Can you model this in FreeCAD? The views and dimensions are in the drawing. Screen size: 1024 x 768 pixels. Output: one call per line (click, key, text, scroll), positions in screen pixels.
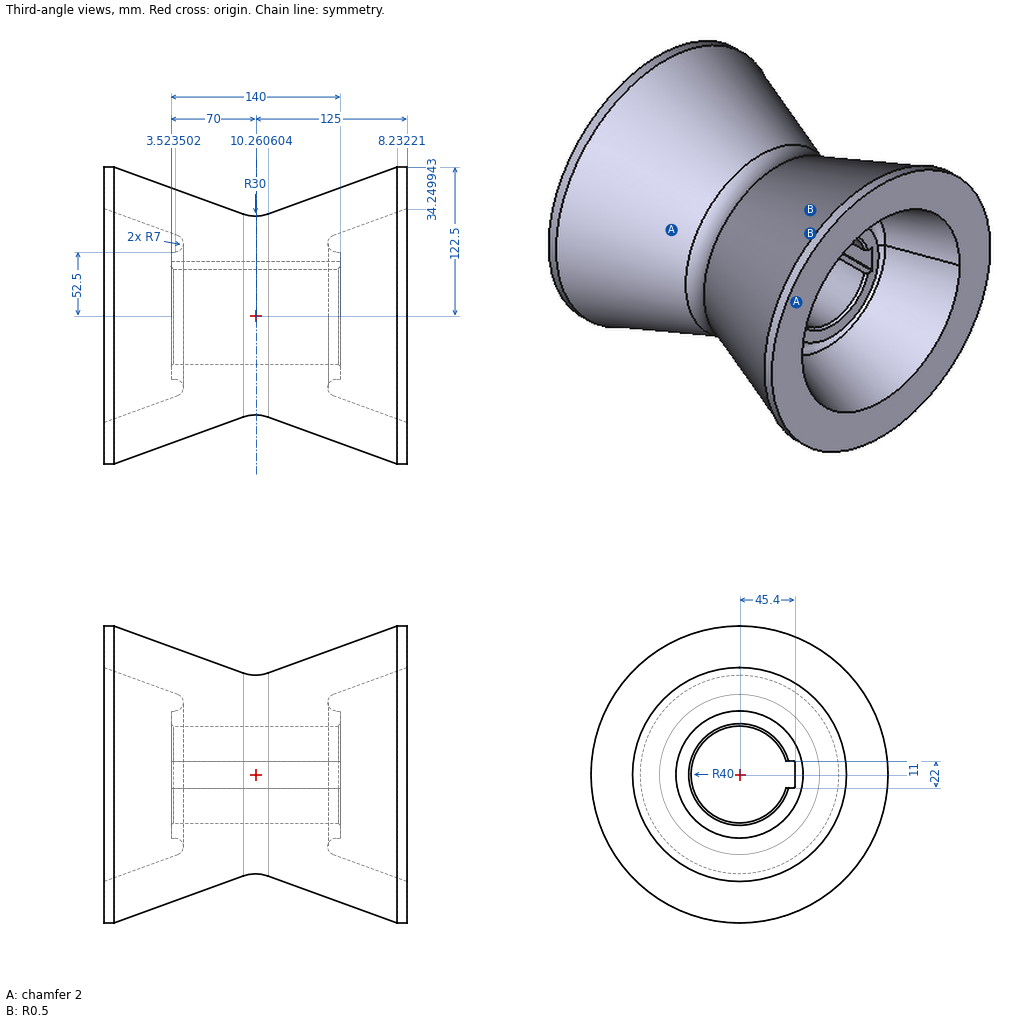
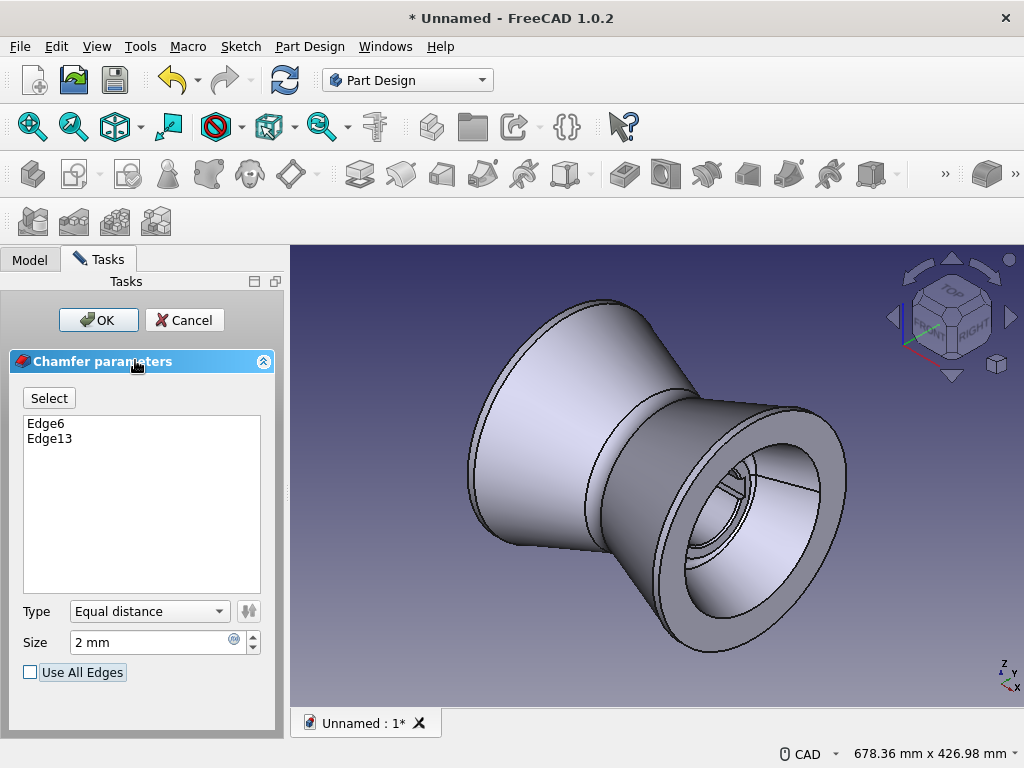
click(99, 320)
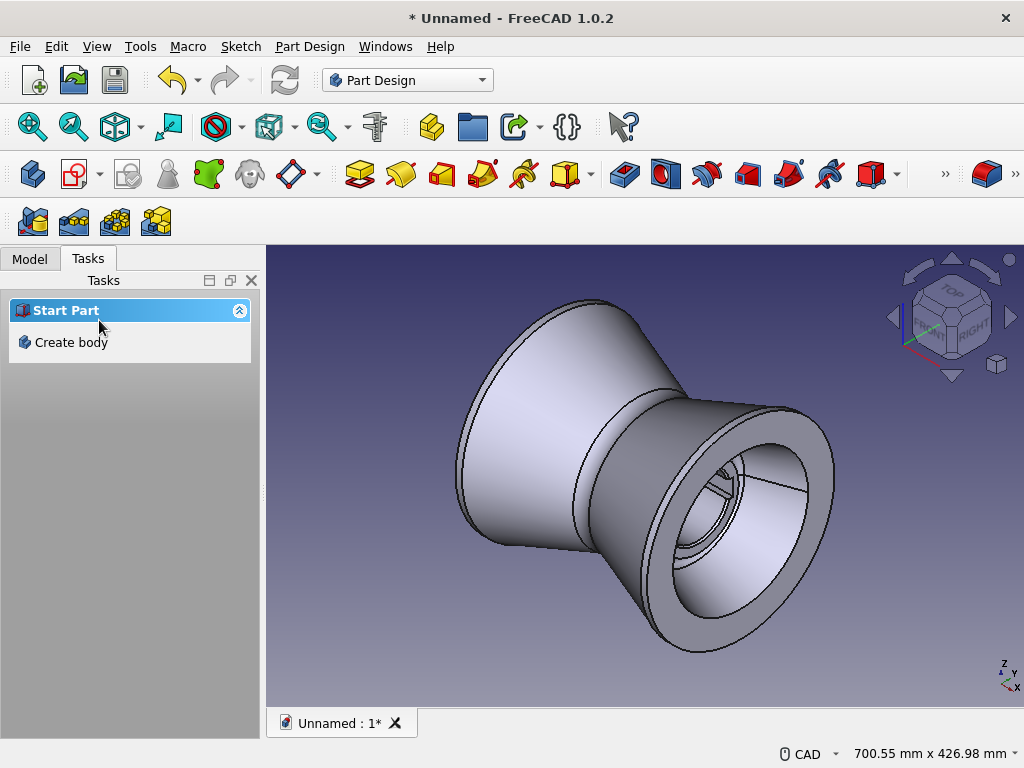
key(2)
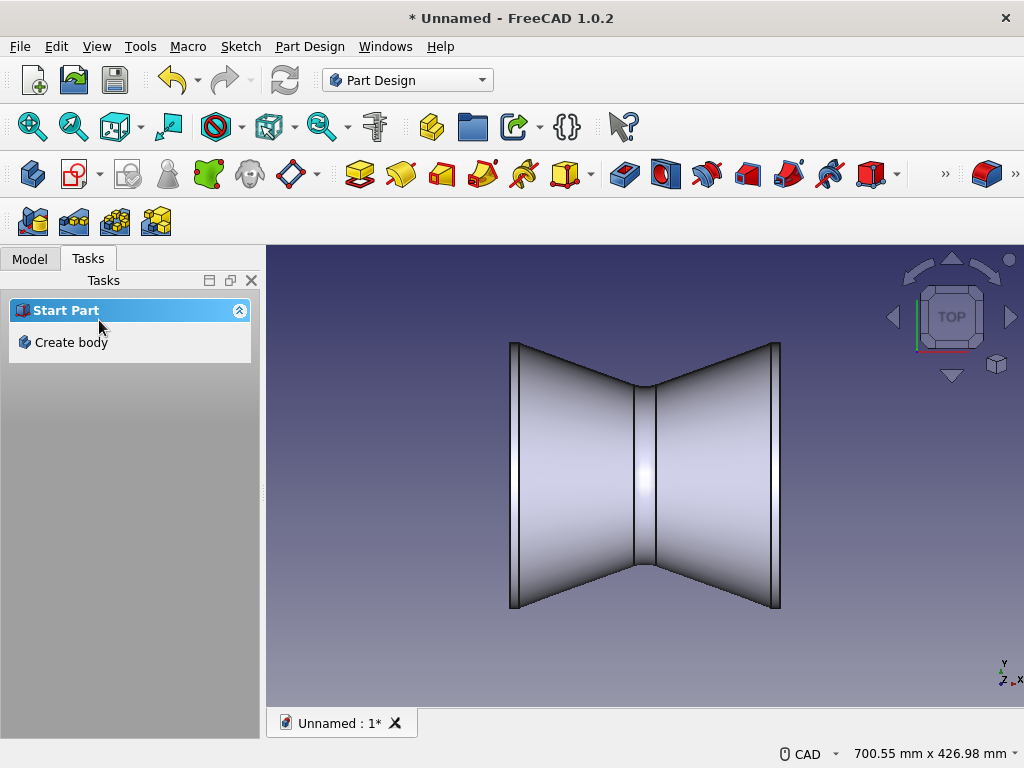
key(0)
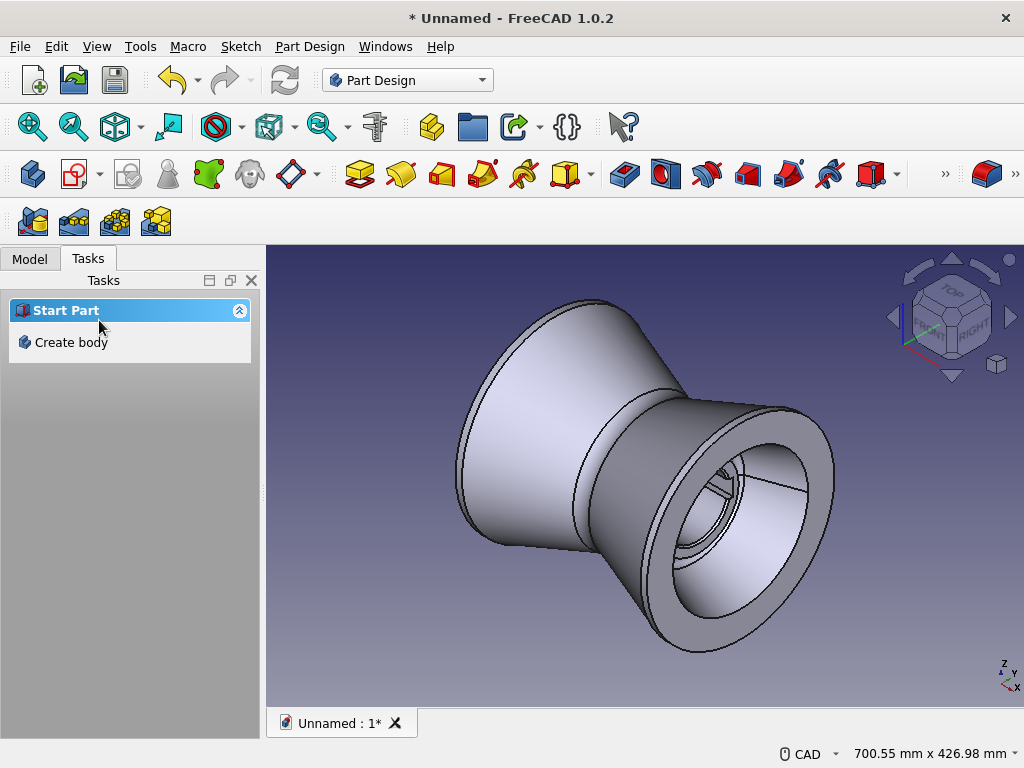
key(1)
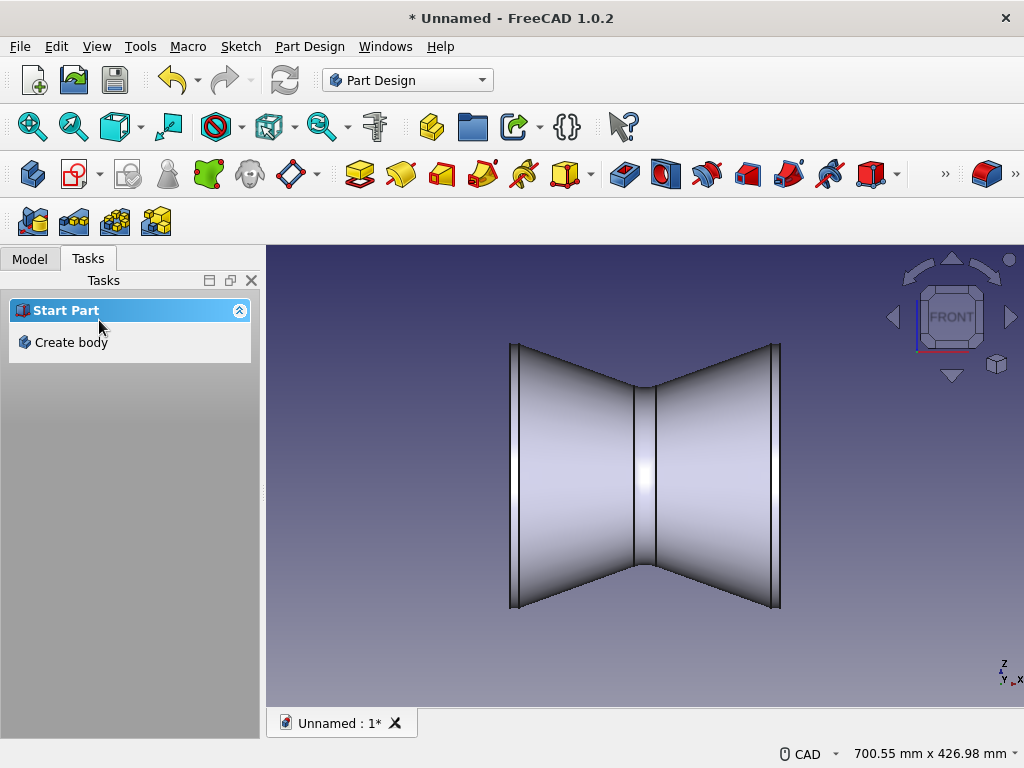
key(3)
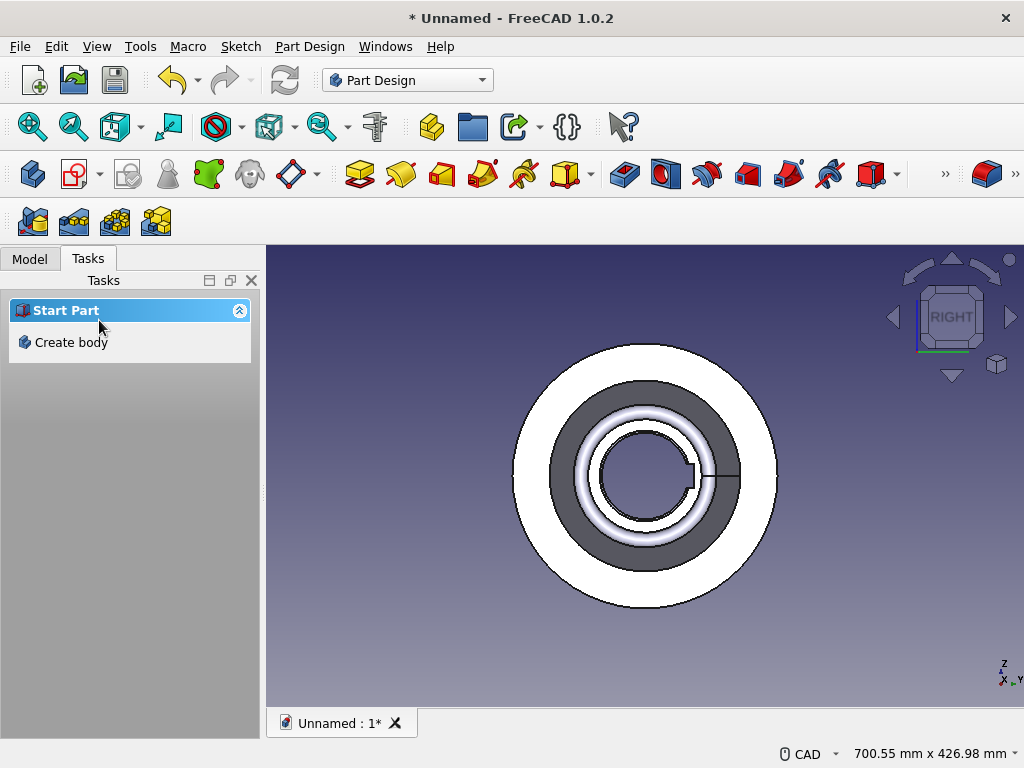
key(5)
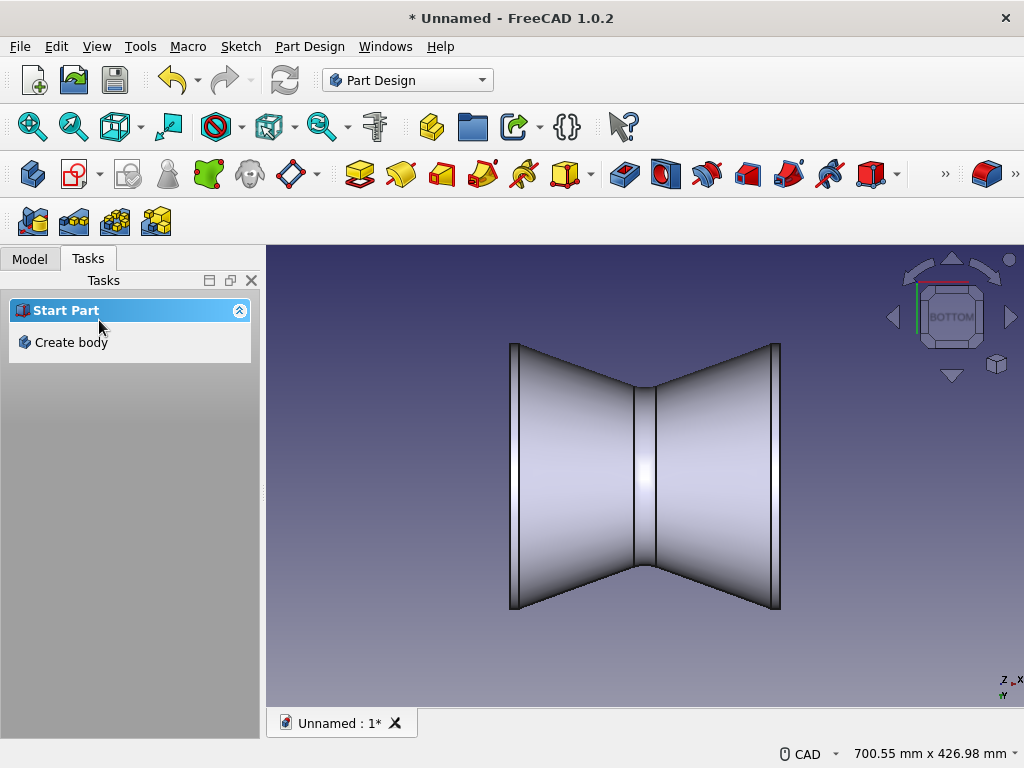
key(4)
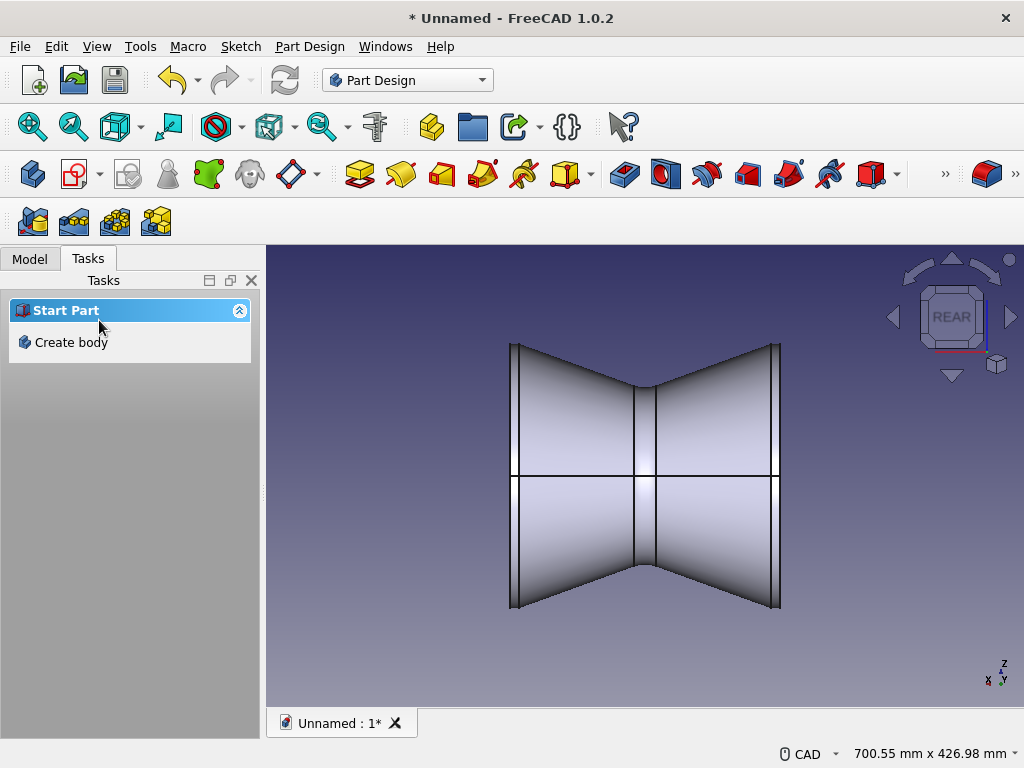
key(6)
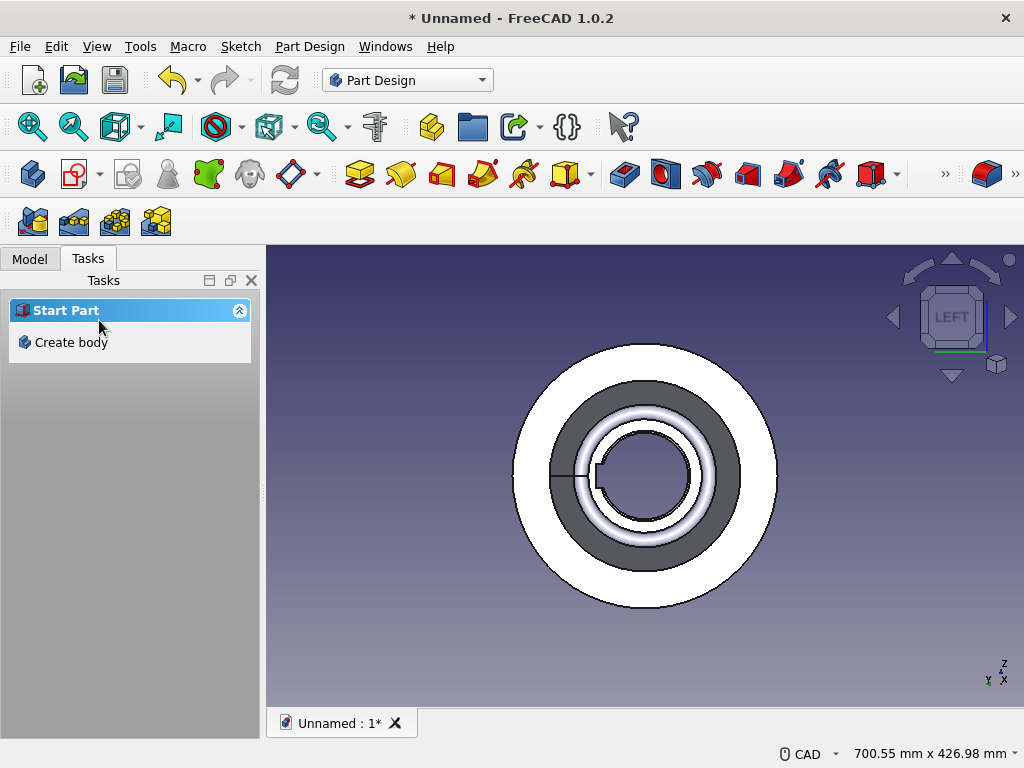
key(v)
key(3)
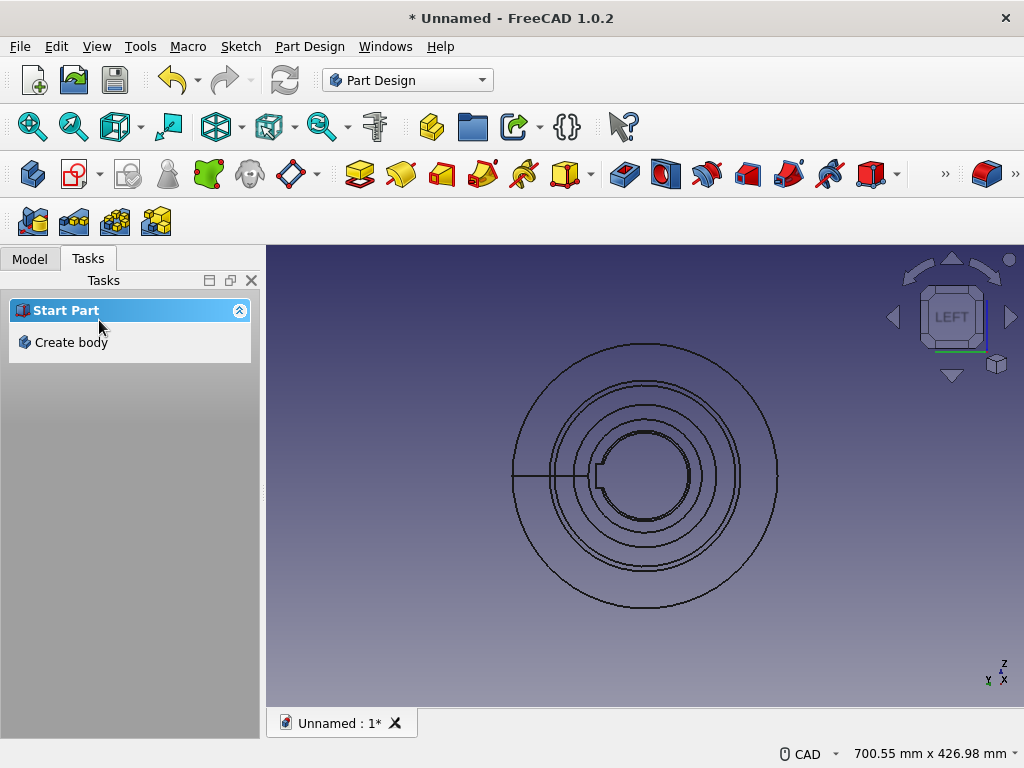
key(0)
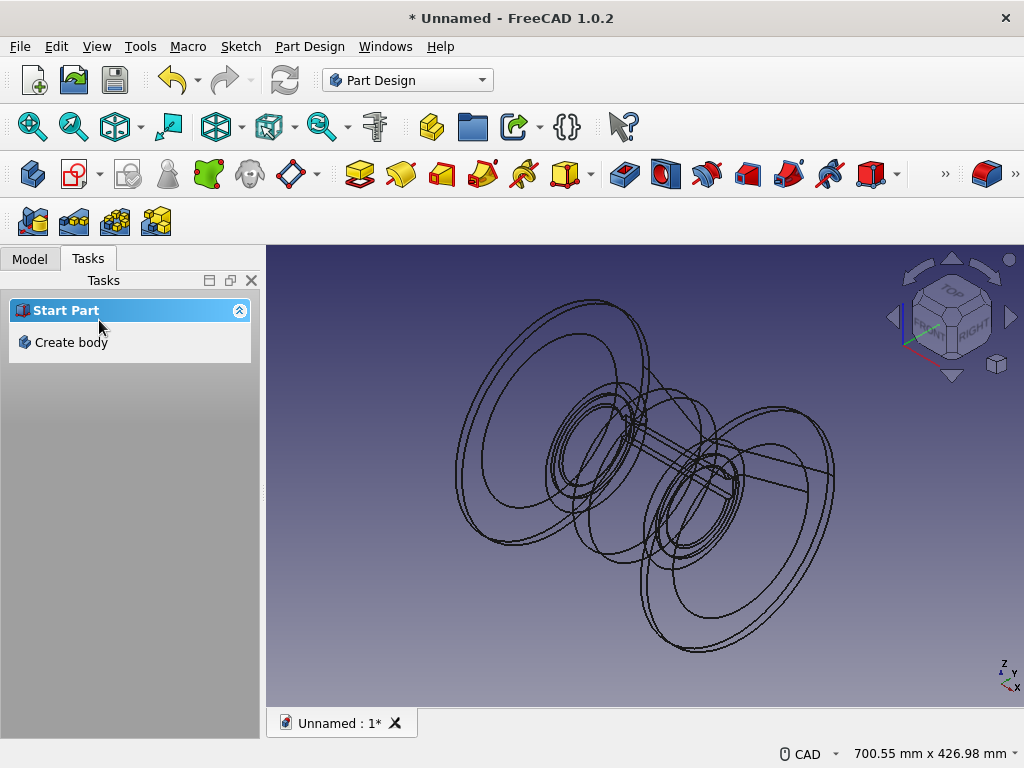
key(2)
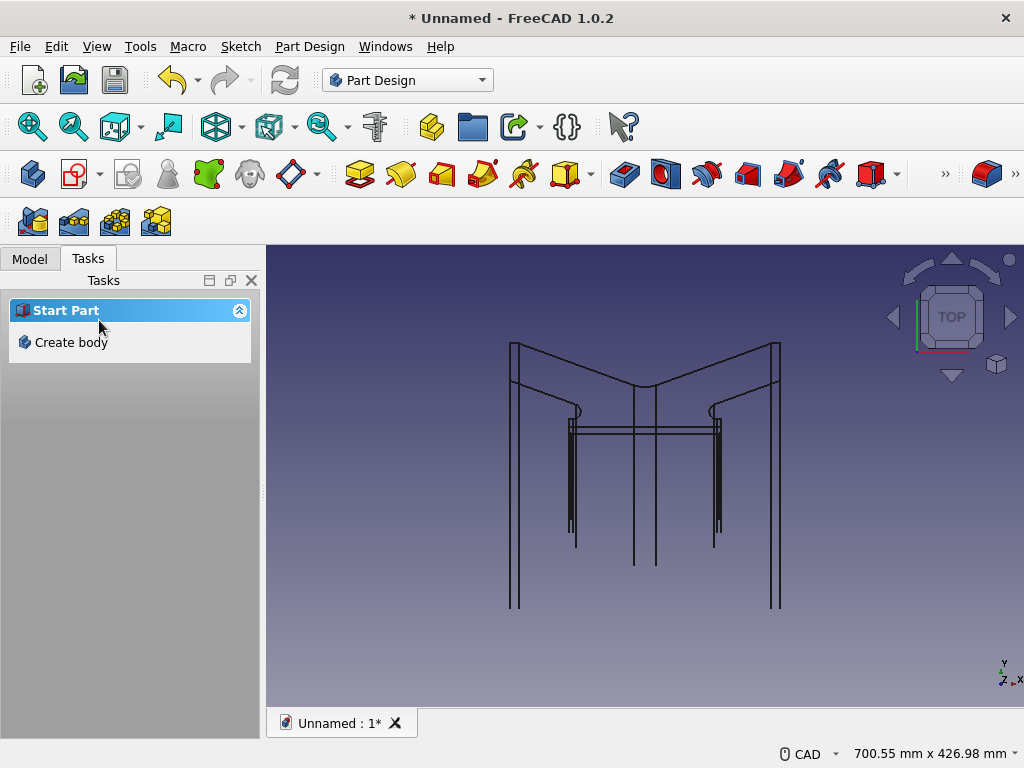
click(645, 426)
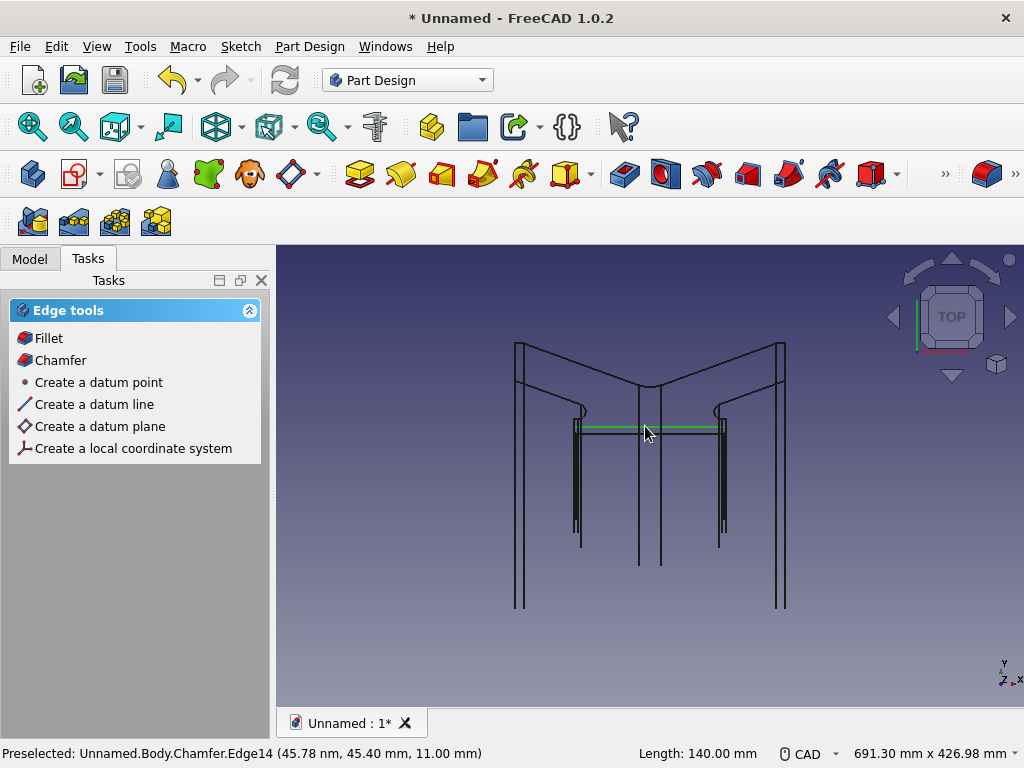
key(1)